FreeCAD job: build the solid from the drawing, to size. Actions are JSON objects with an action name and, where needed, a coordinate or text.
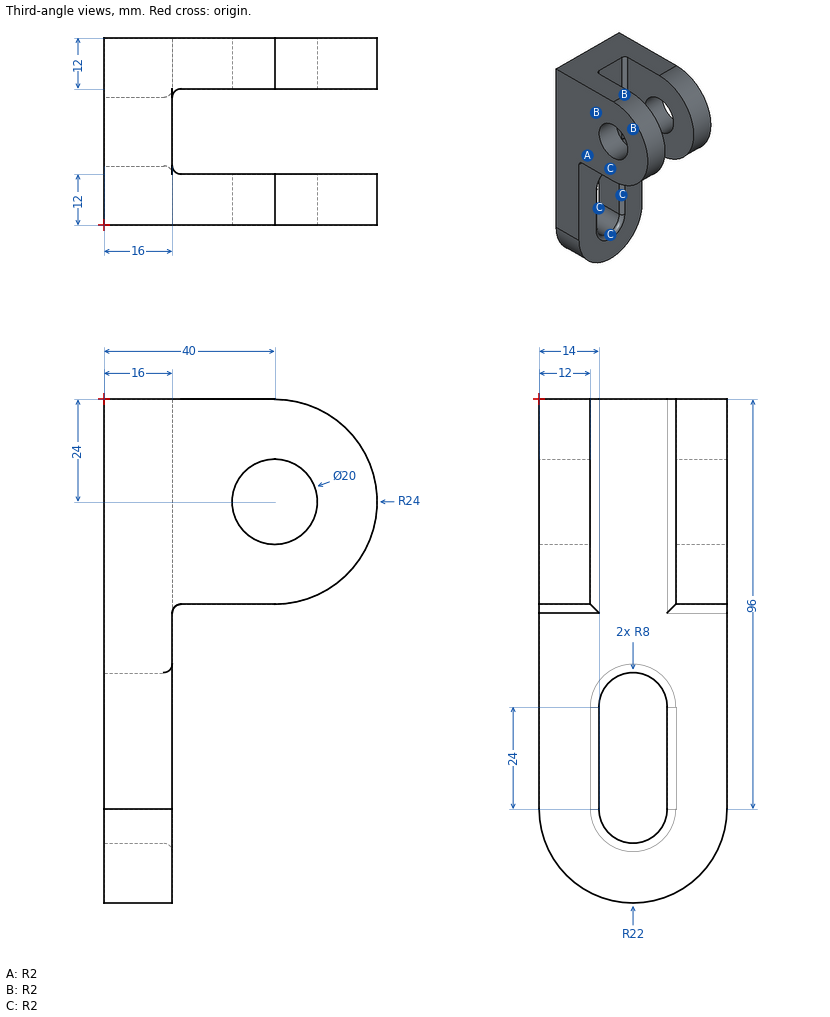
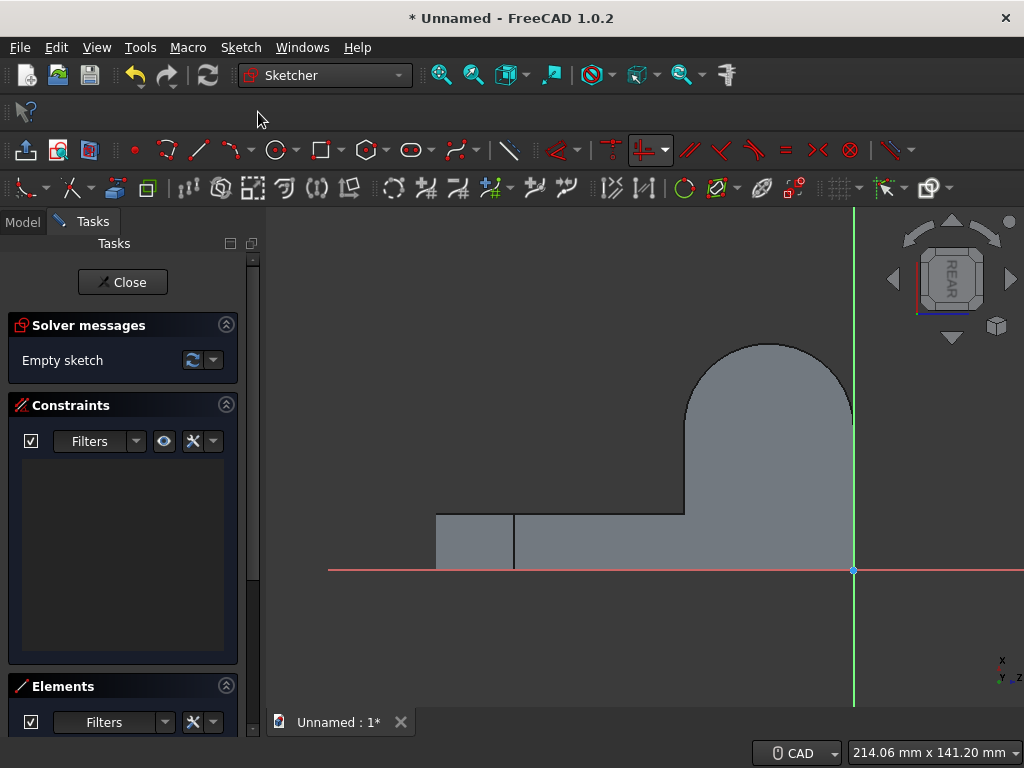
{"action": "scroll", "coordinate": [832, 419], "scroll_direction": "up", "scroll_amount": 7}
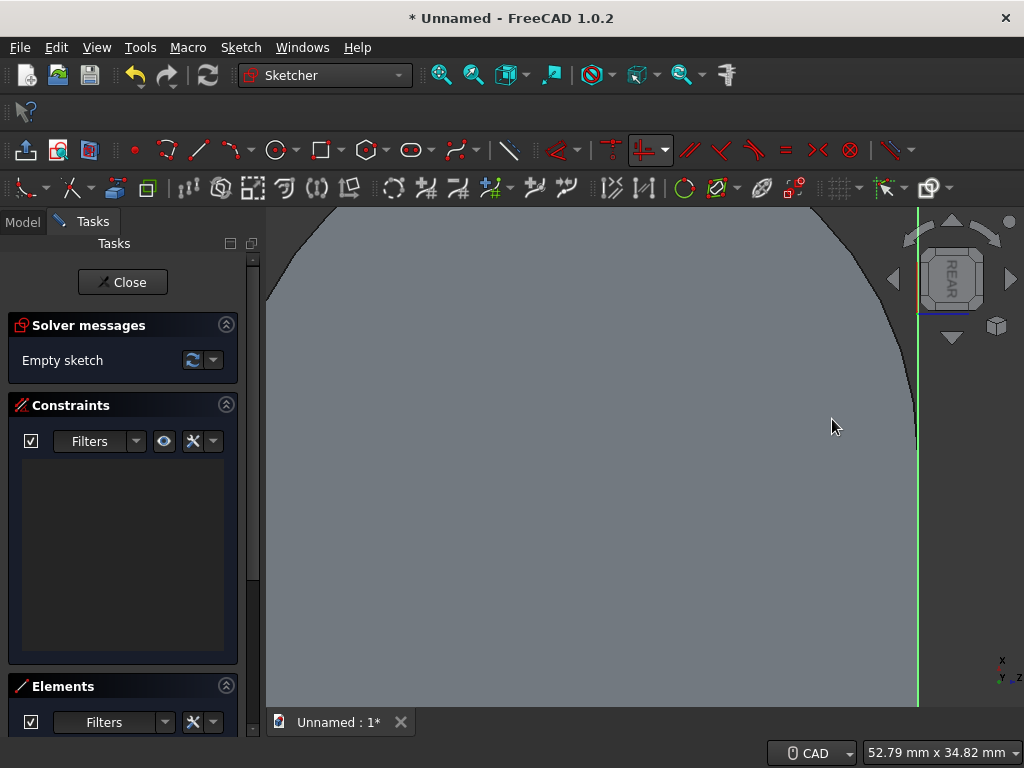
{"action": "left_click", "coordinate": [276, 150]}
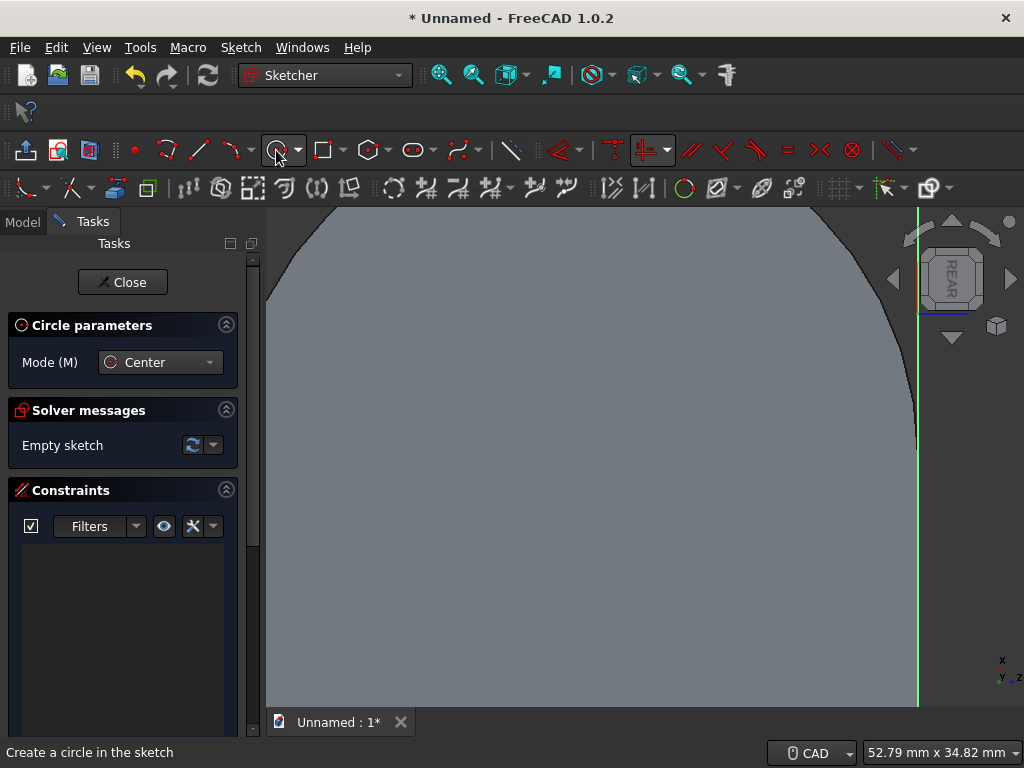
{"action": "left_click", "coordinate": [573, 457]}
{"action": "mouse_move", "coordinate": [675, 355]}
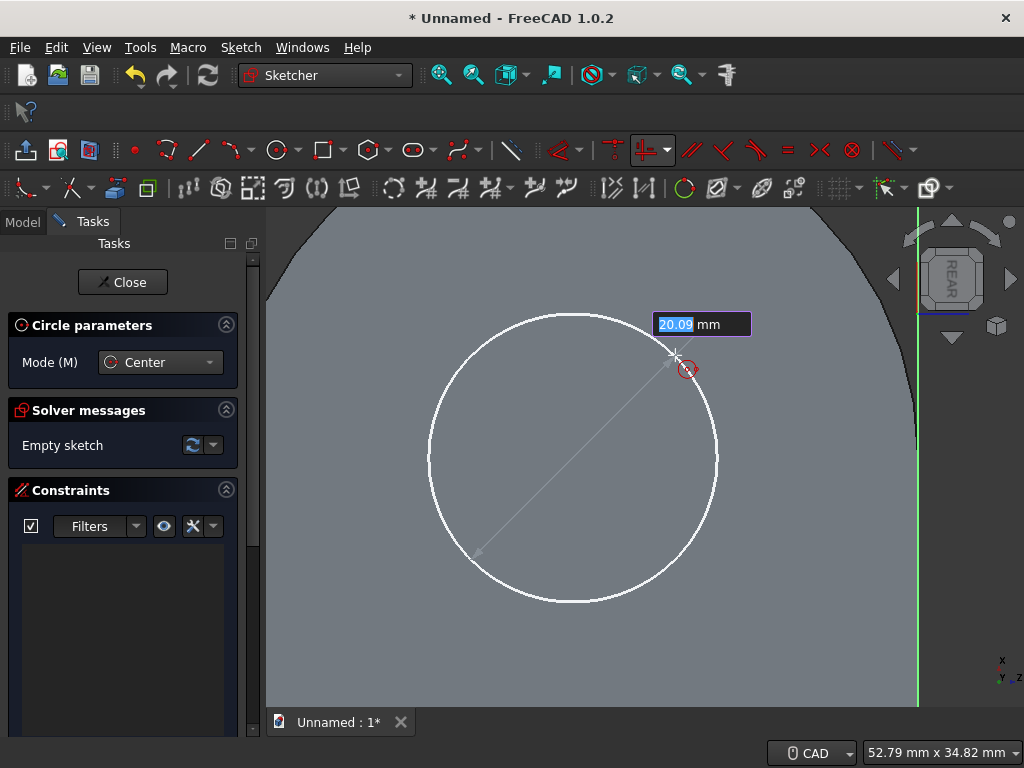
{"action": "type", "text": "20"}
{"action": "key", "text": "Return"}
{"action": "key", "text": "Escape"}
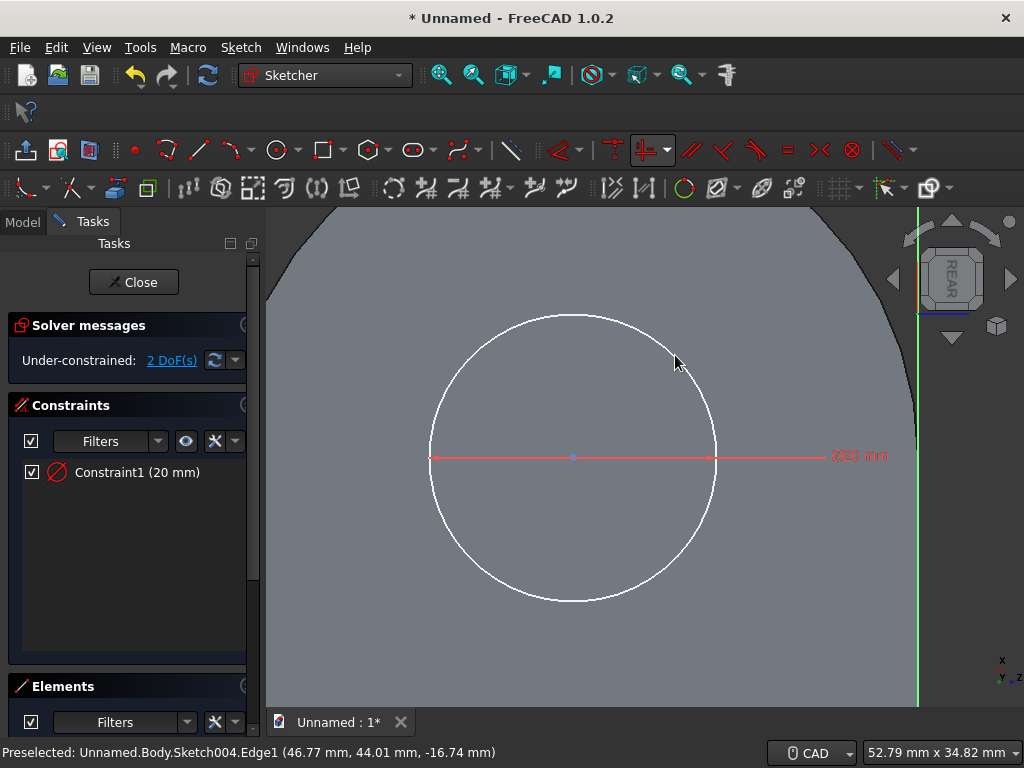
{"action": "left_click", "coordinate": [558, 150]}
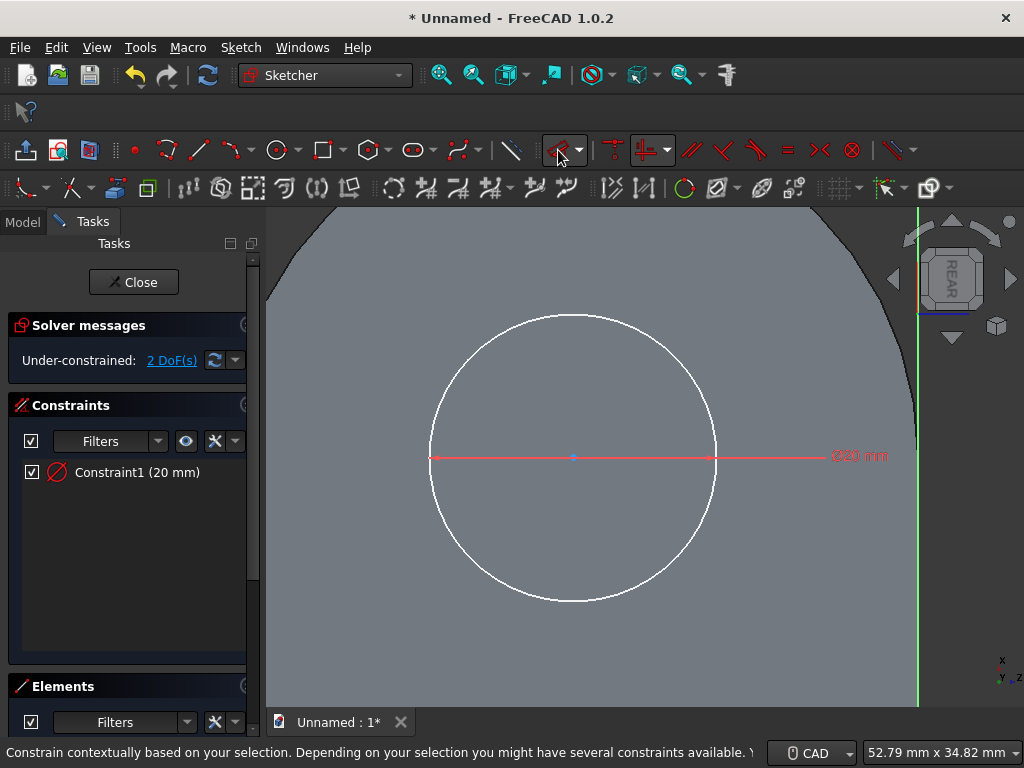
{"action": "left_click", "coordinate": [573, 458]}
{"action": "left_click", "coordinate": [650, 424]}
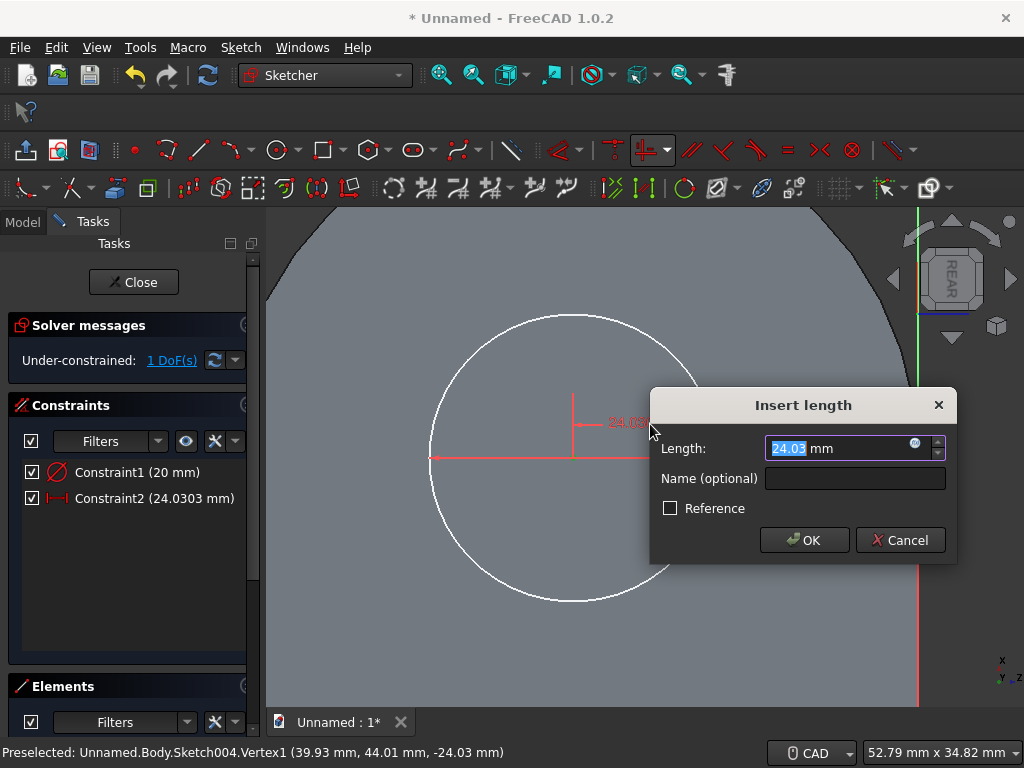
{"action": "type", "text": "24"}
{"action": "key", "text": "Return"}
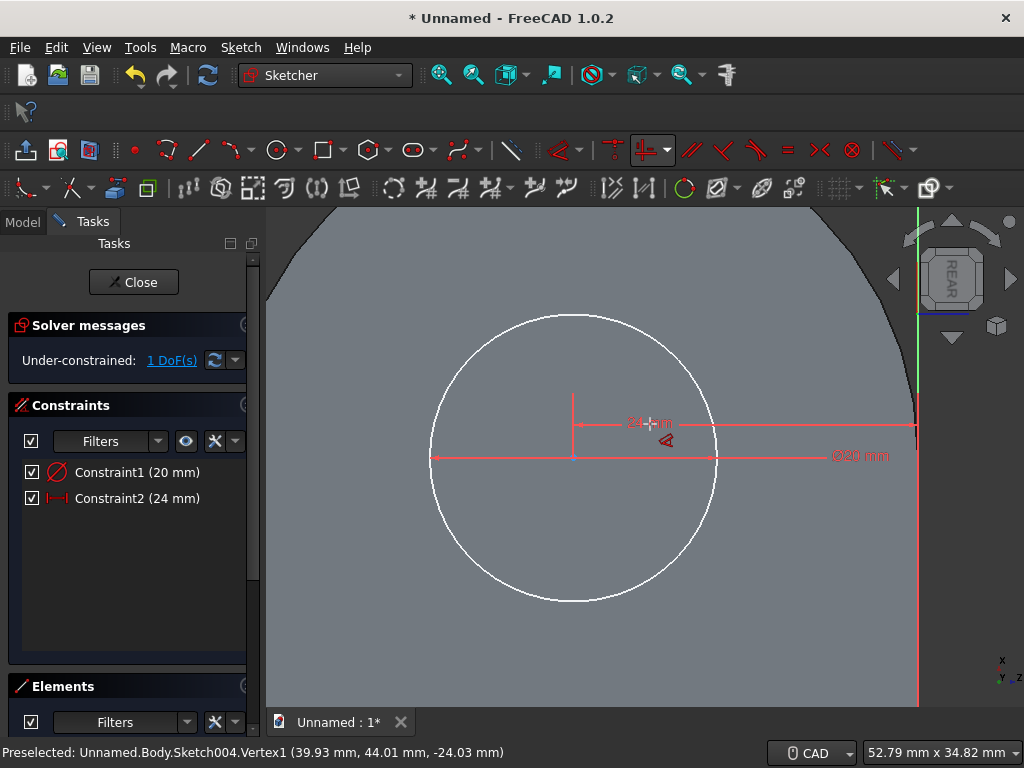
{"action": "left_click", "coordinate": [573, 458]}
{"action": "left_click", "coordinate": [539, 569]}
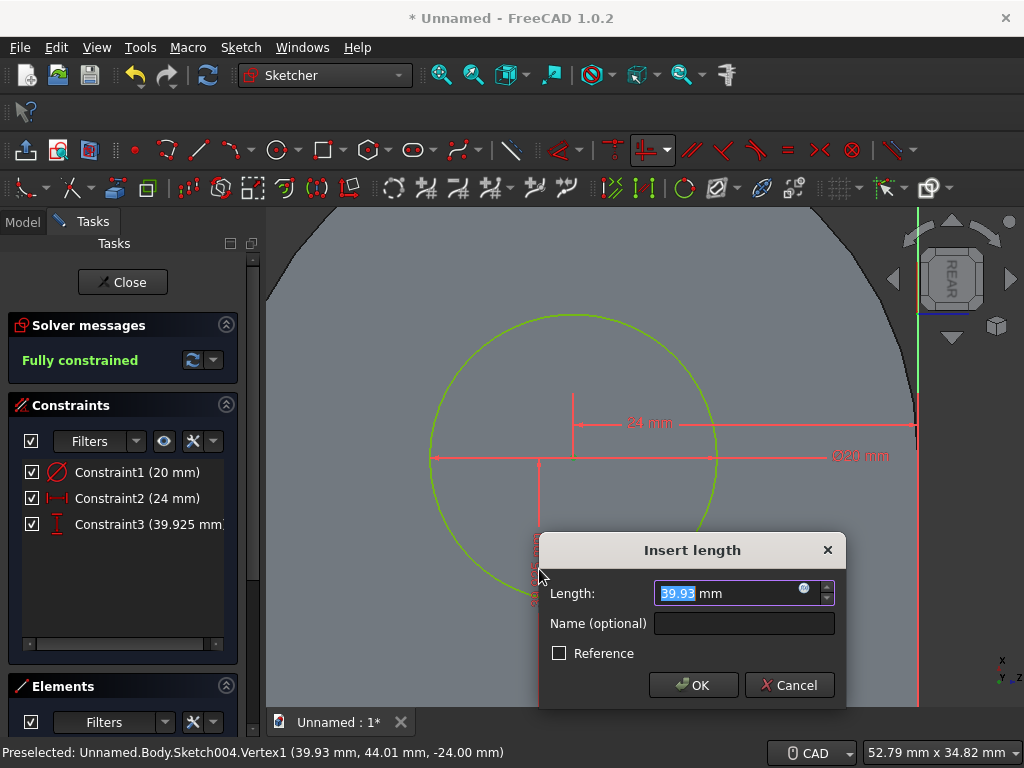
{"action": "type", "text": "40"}
{"action": "key", "text": "Return"}
{"action": "key", "text": "Escape"}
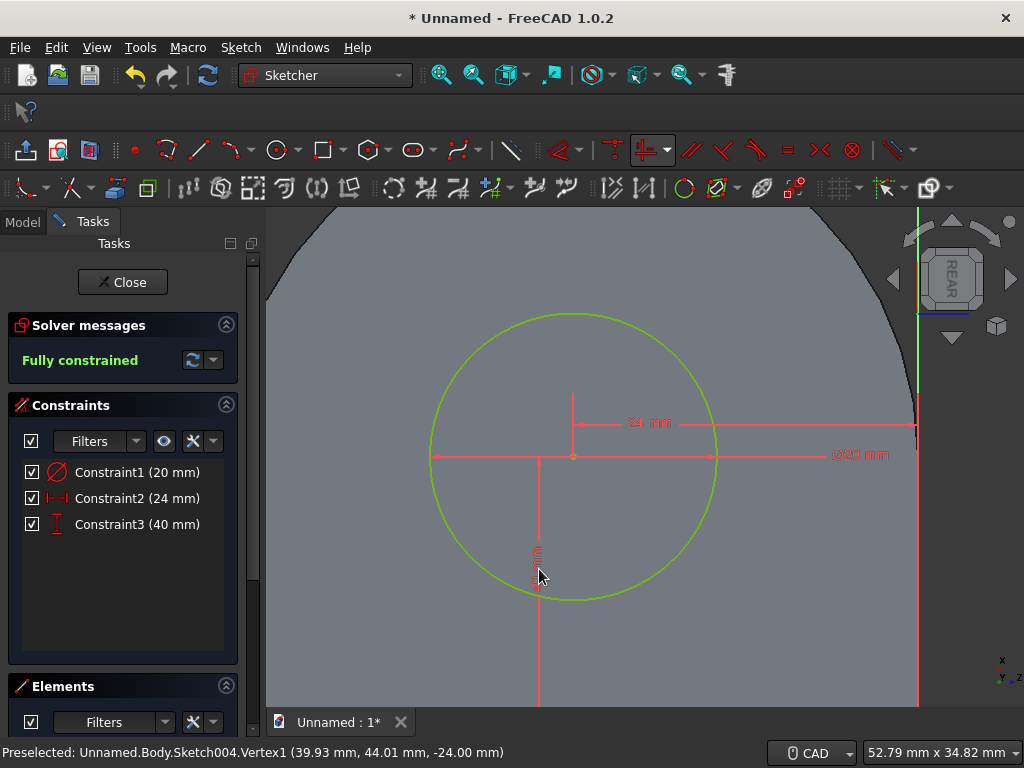
{"action": "left_click", "coordinate": [123, 282]}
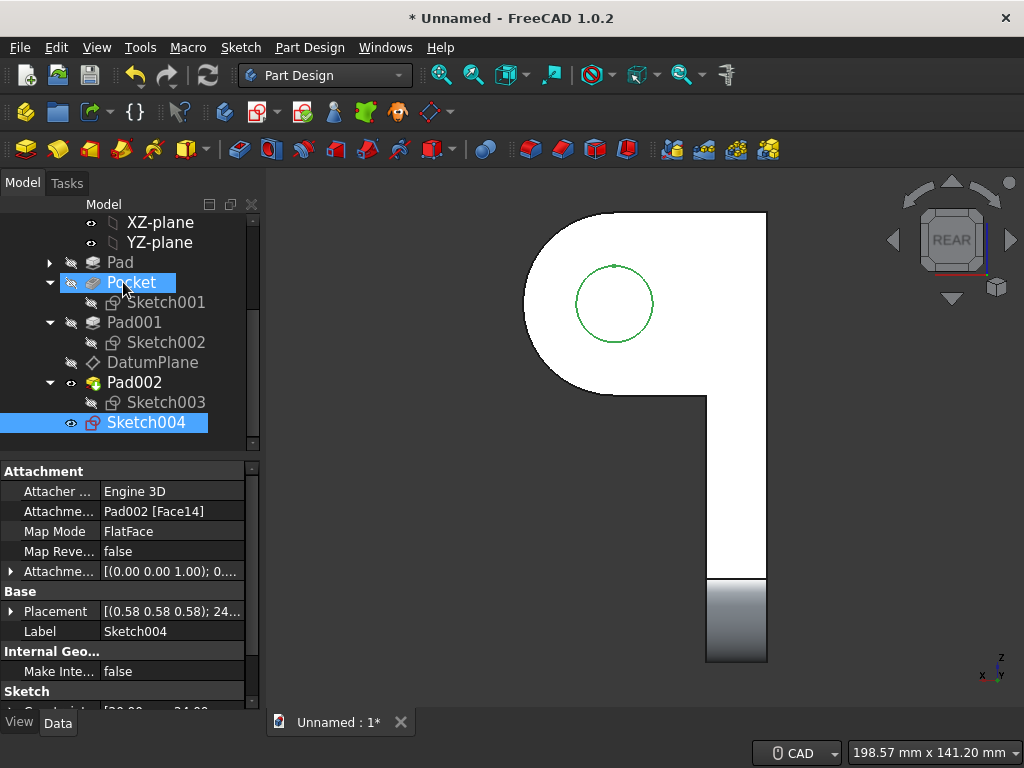
{"action": "left_click", "coordinate": [240, 150]}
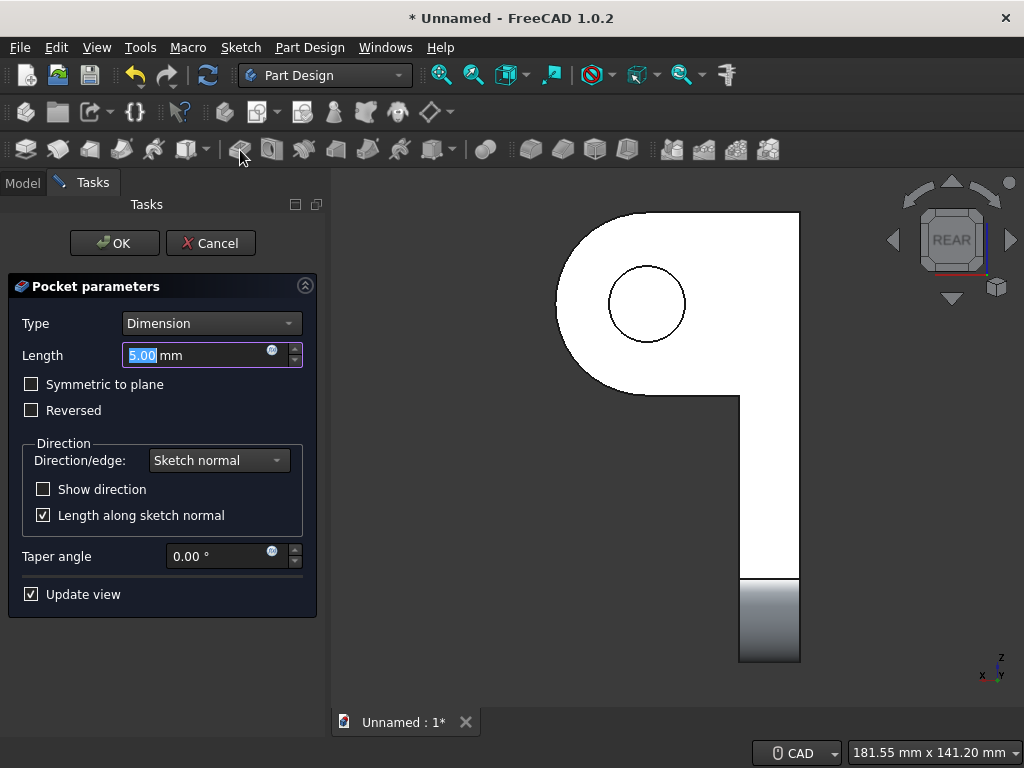
{"action": "type", "text": "12"}
{"action": "key", "text": "Tab"}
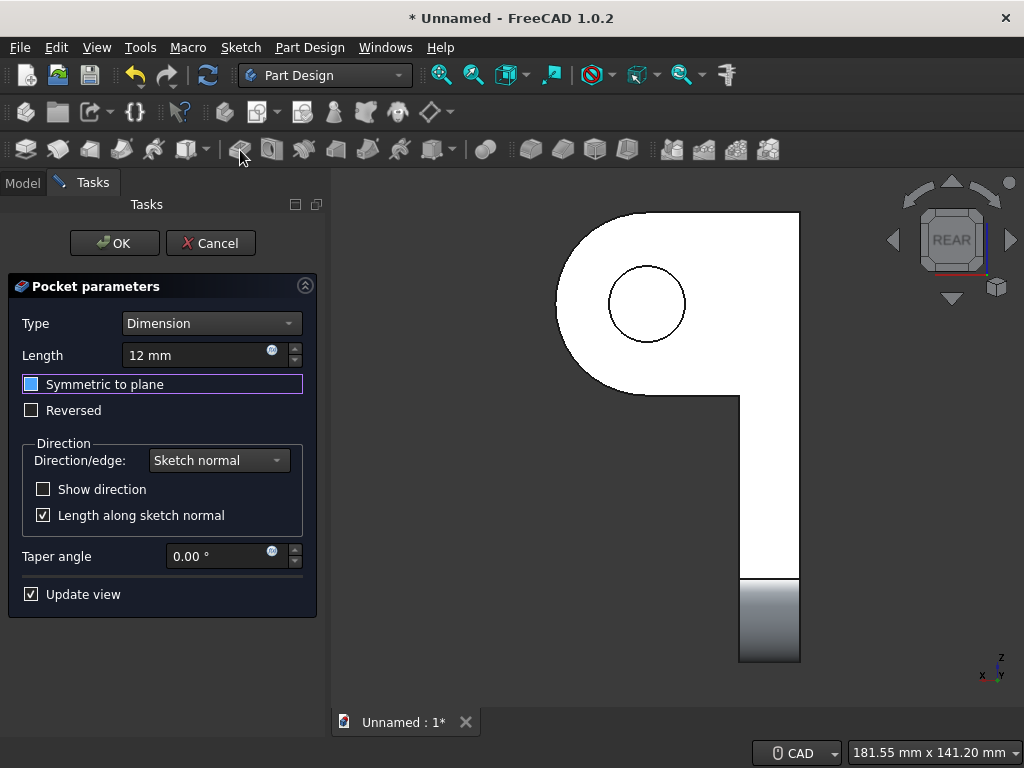
{"action": "left_click", "coordinate": [115, 243]}